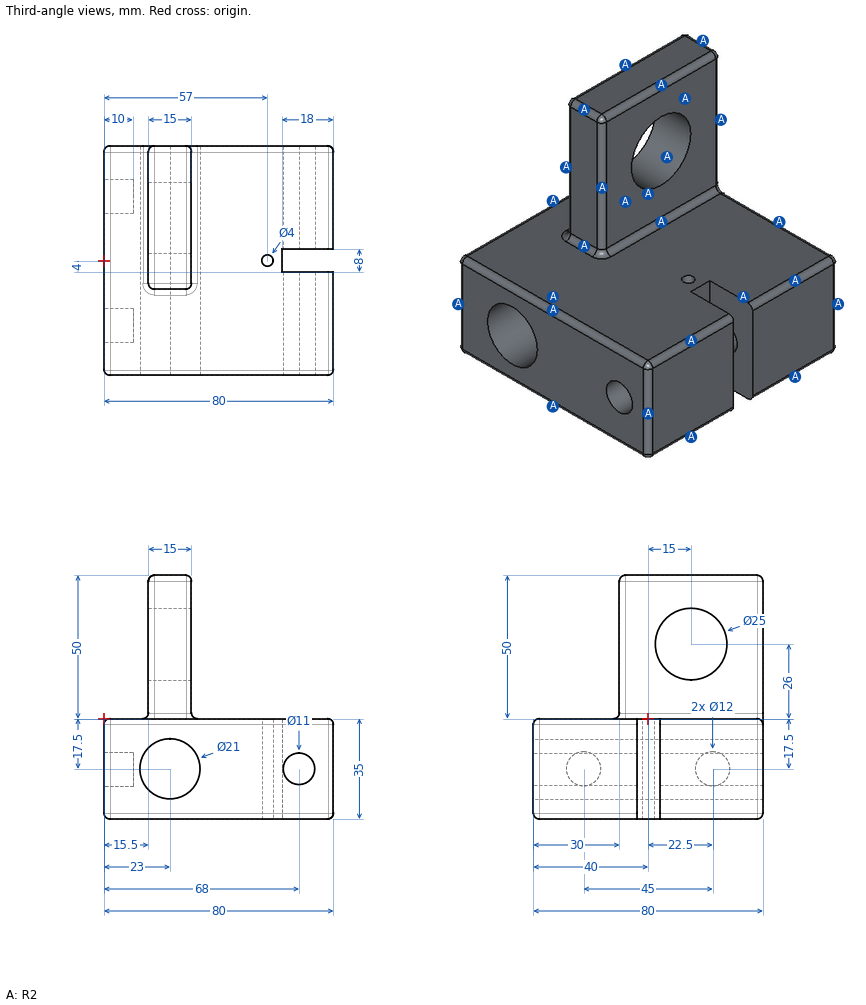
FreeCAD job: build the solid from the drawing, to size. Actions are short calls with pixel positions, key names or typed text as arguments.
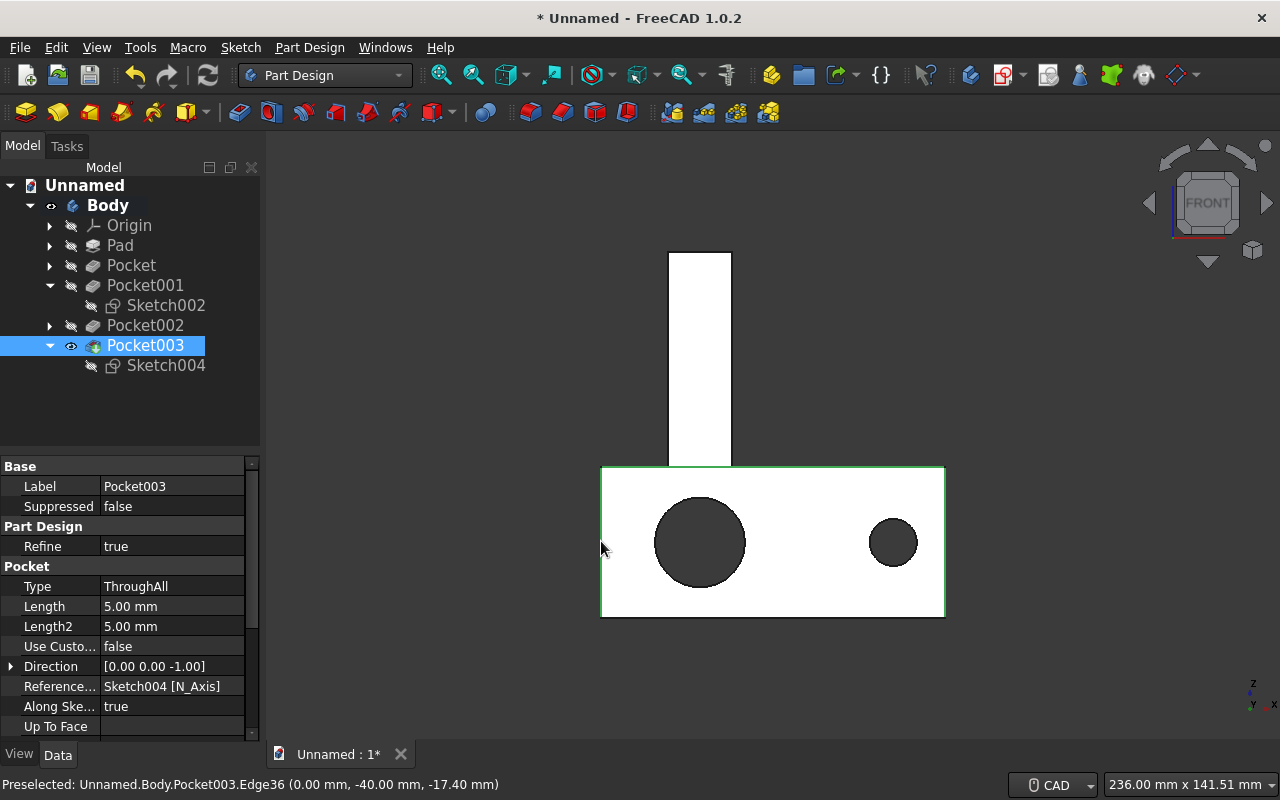
click(945, 541, ctrl)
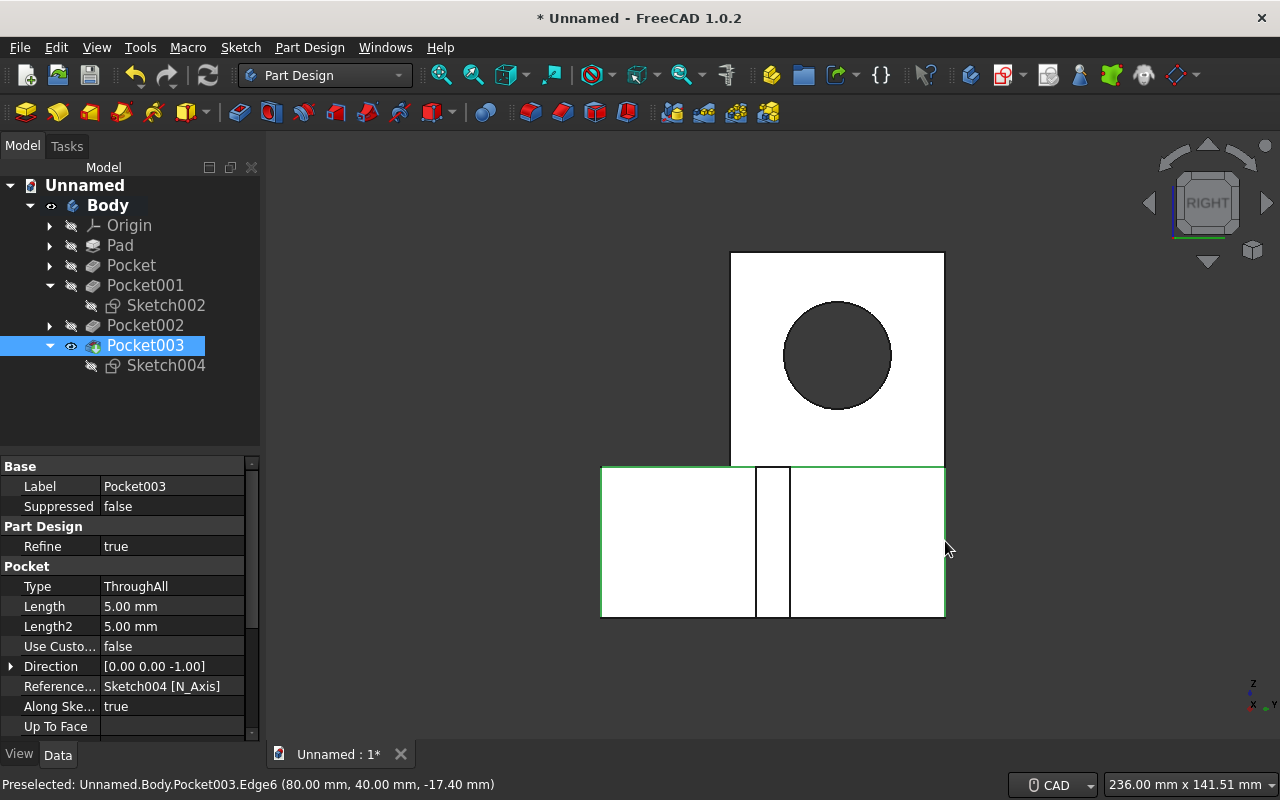
click(868, 617, ctrl)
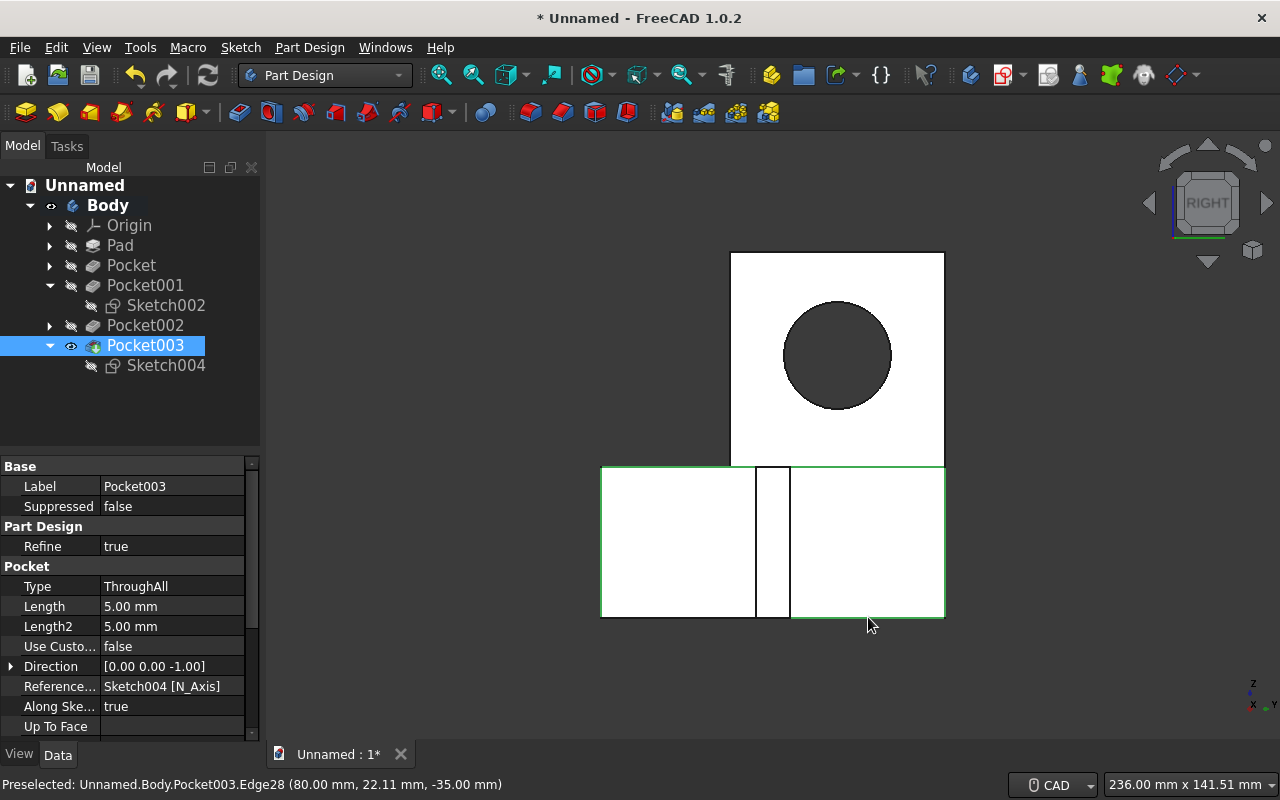
click(945, 359, ctrl)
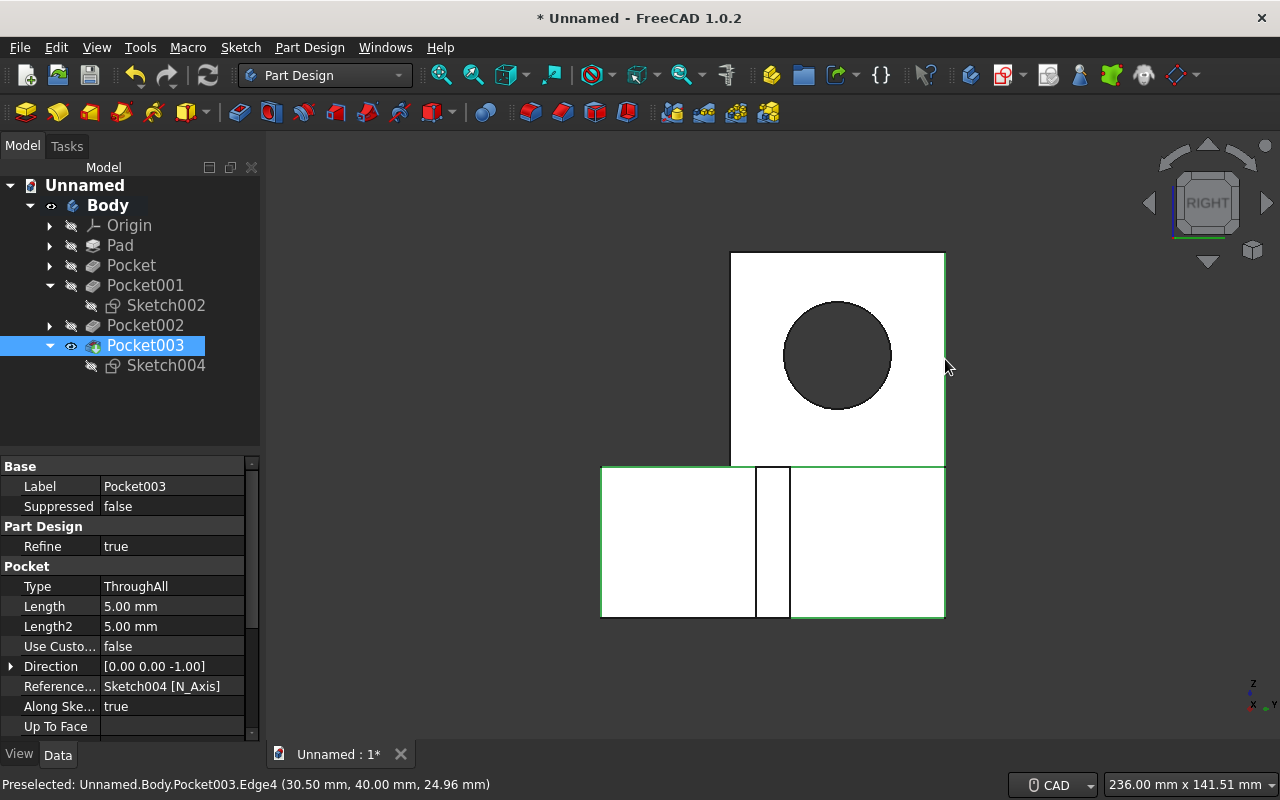
click(678, 617, ctrl)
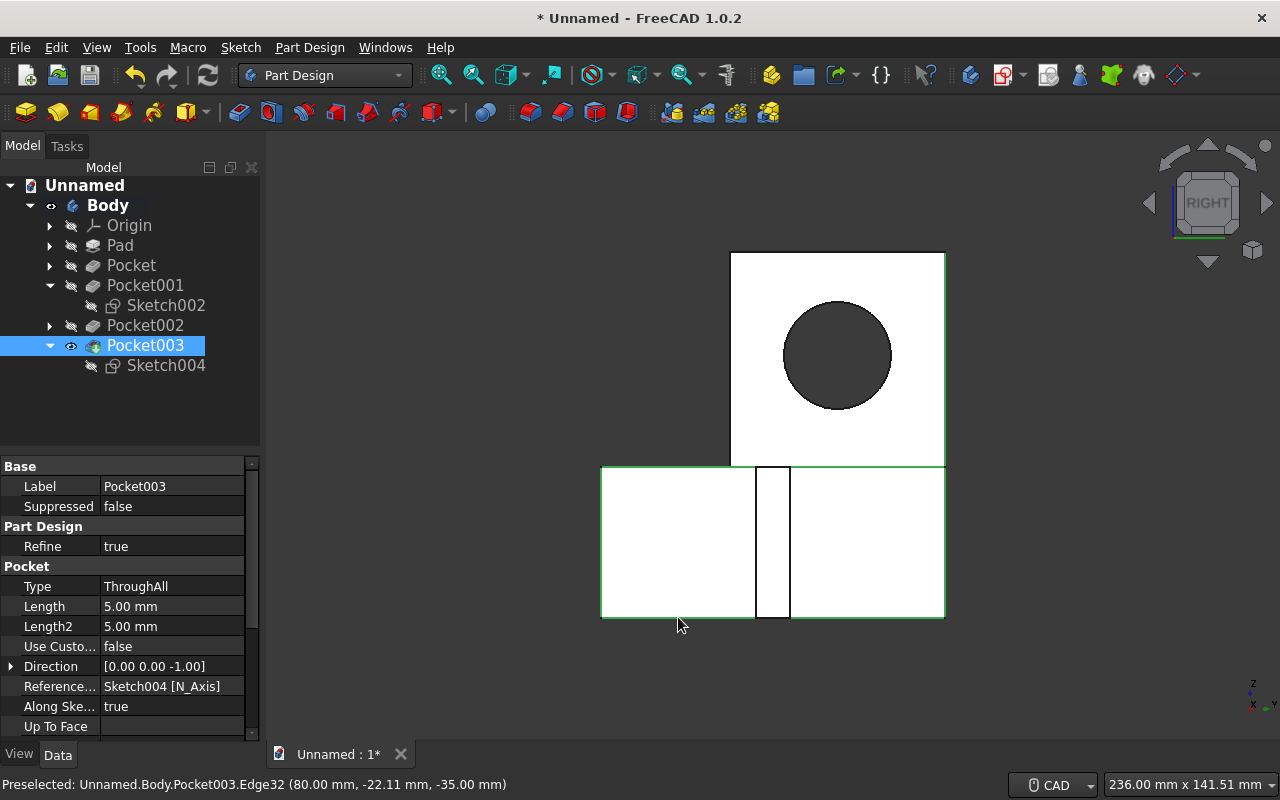
key(5)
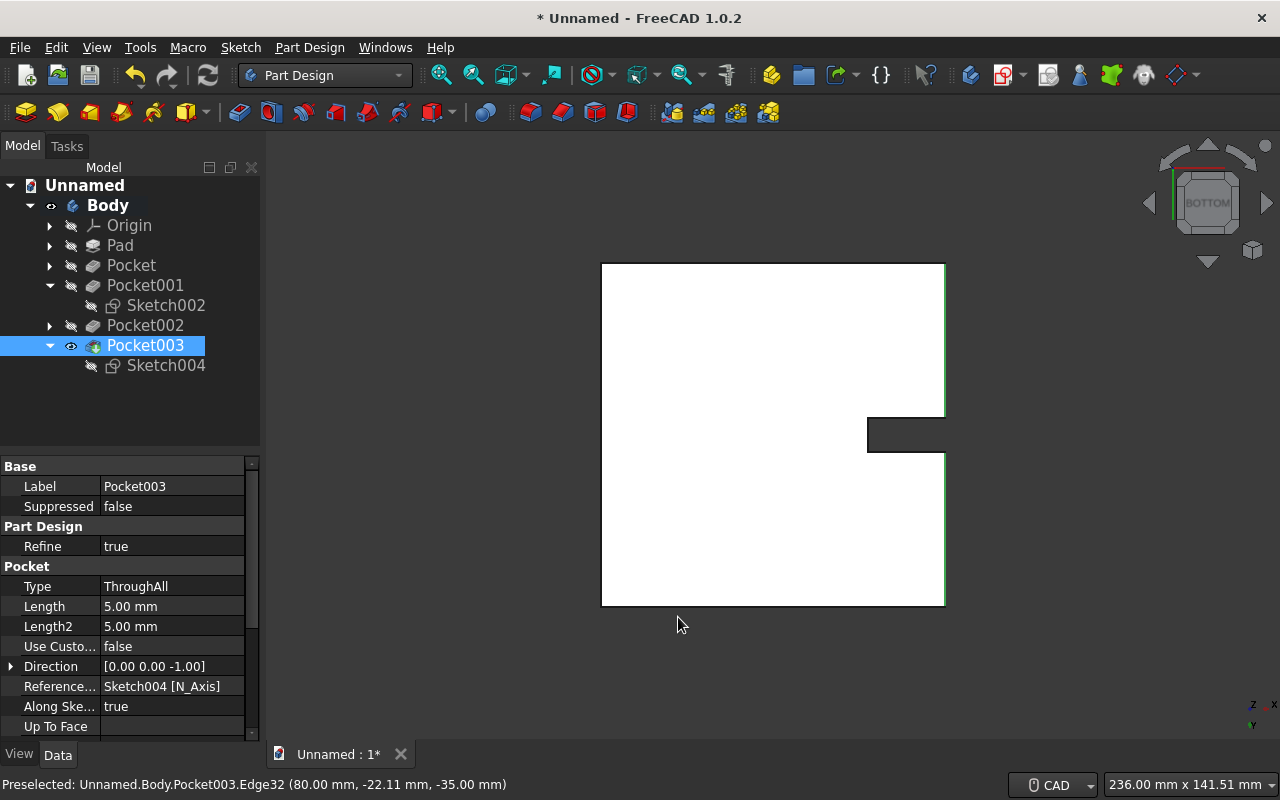
click(773, 262, ctrl)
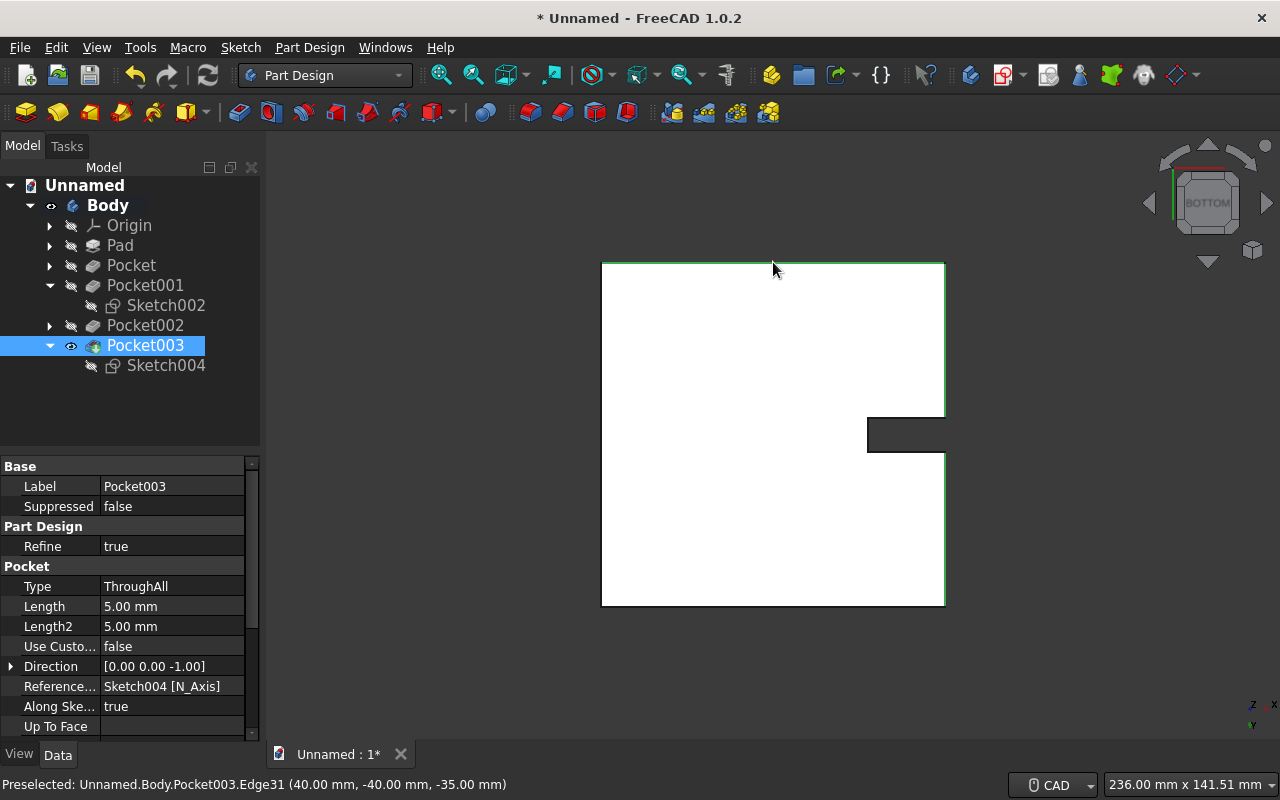
click(601, 434, ctrl)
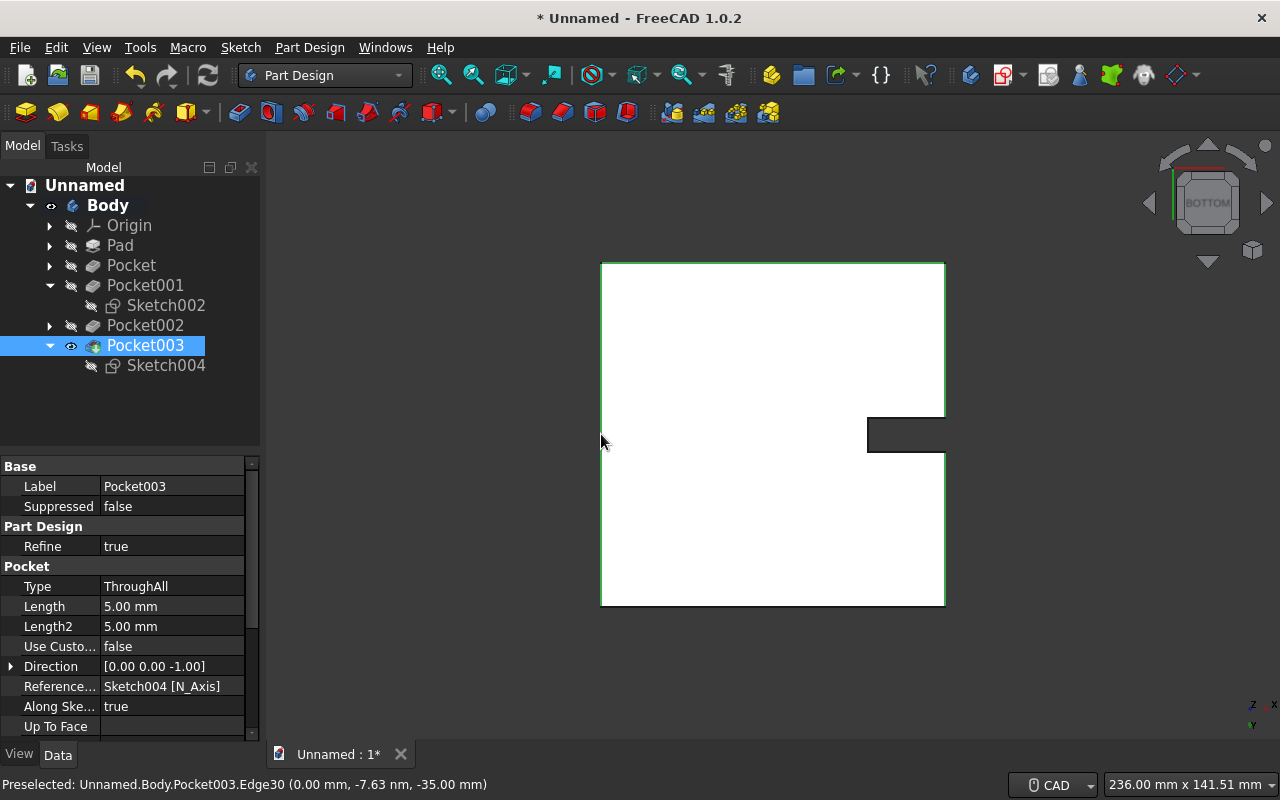
key(4)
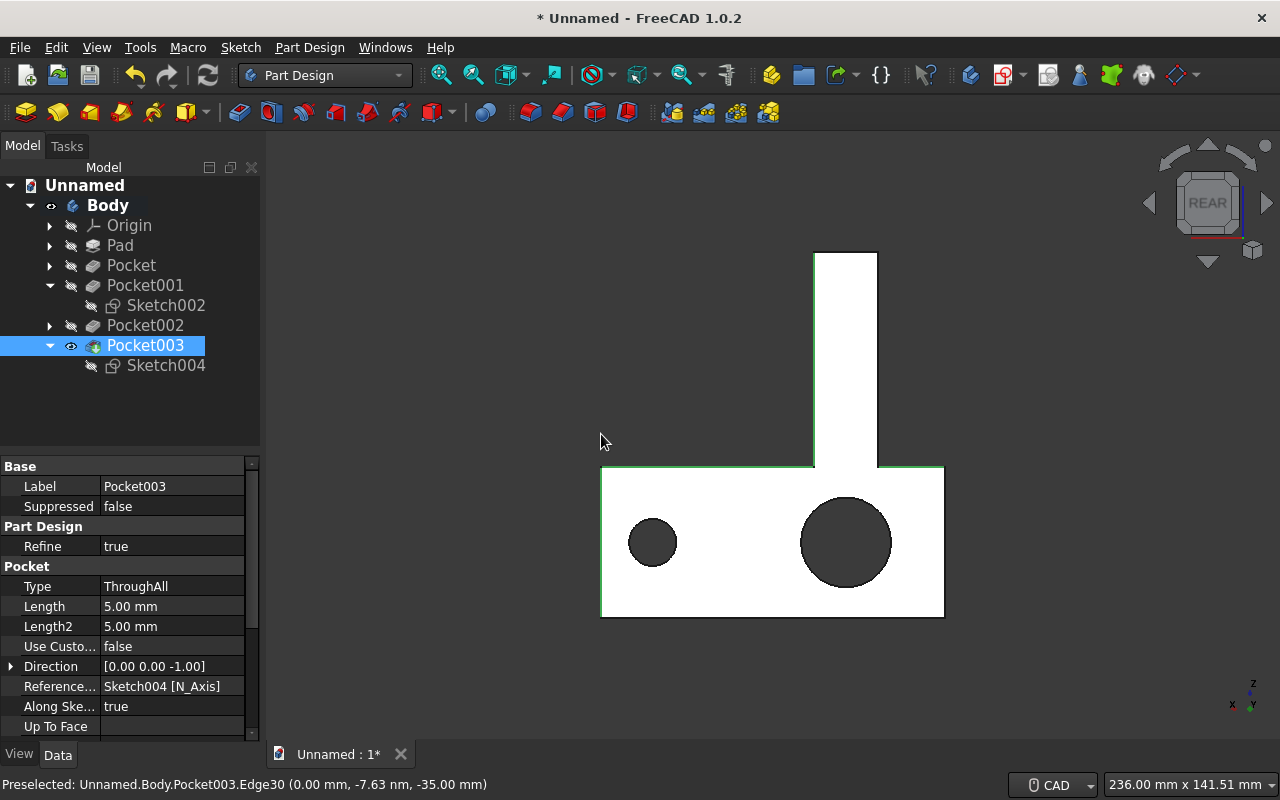
click(773, 617, ctrl)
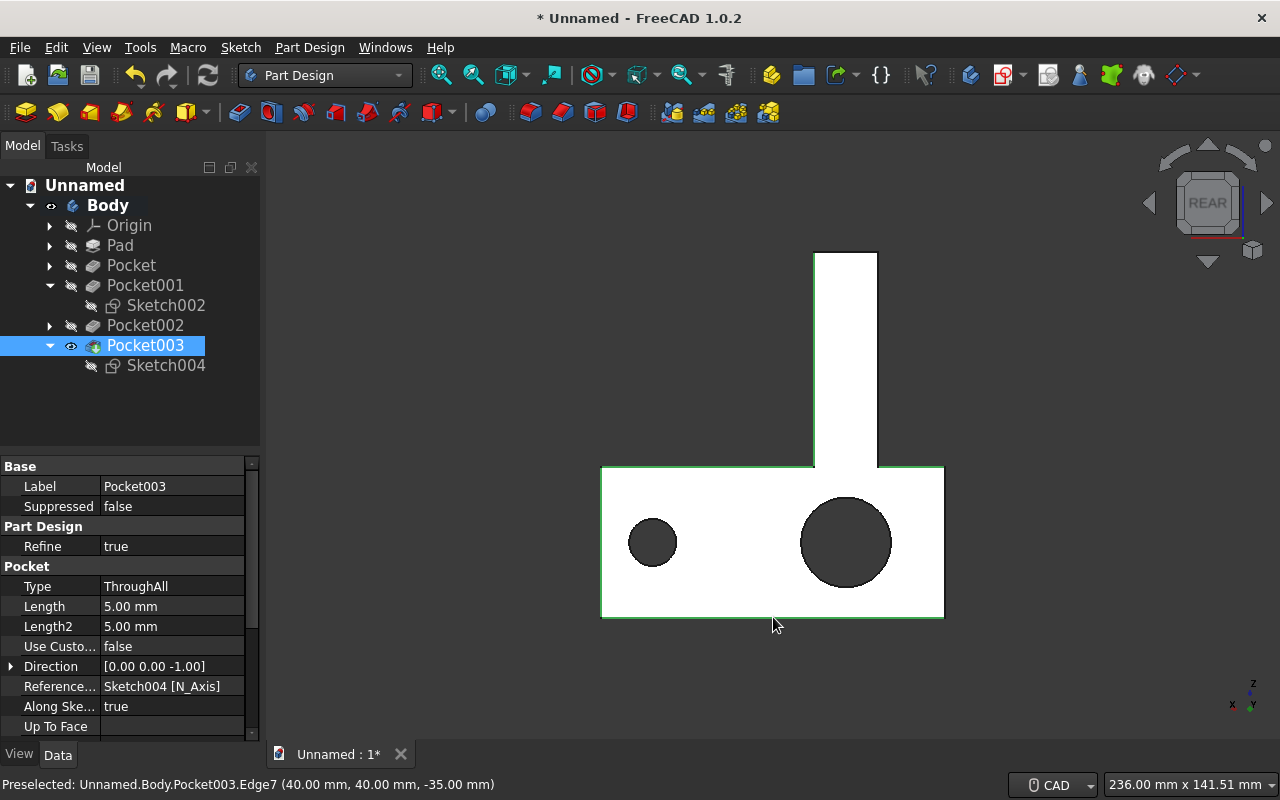
click(945, 541, ctrl)